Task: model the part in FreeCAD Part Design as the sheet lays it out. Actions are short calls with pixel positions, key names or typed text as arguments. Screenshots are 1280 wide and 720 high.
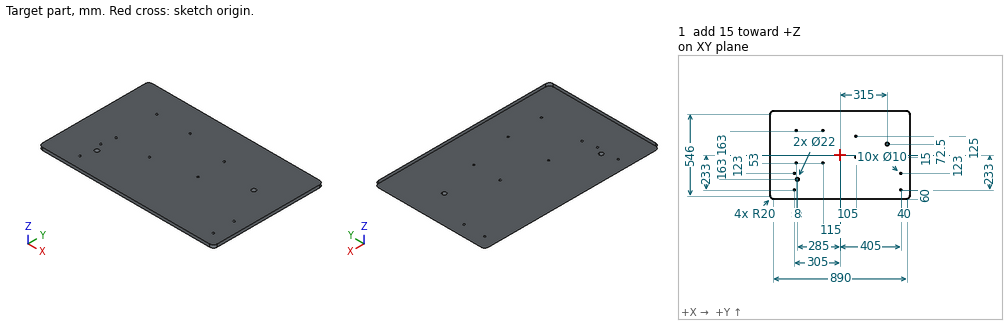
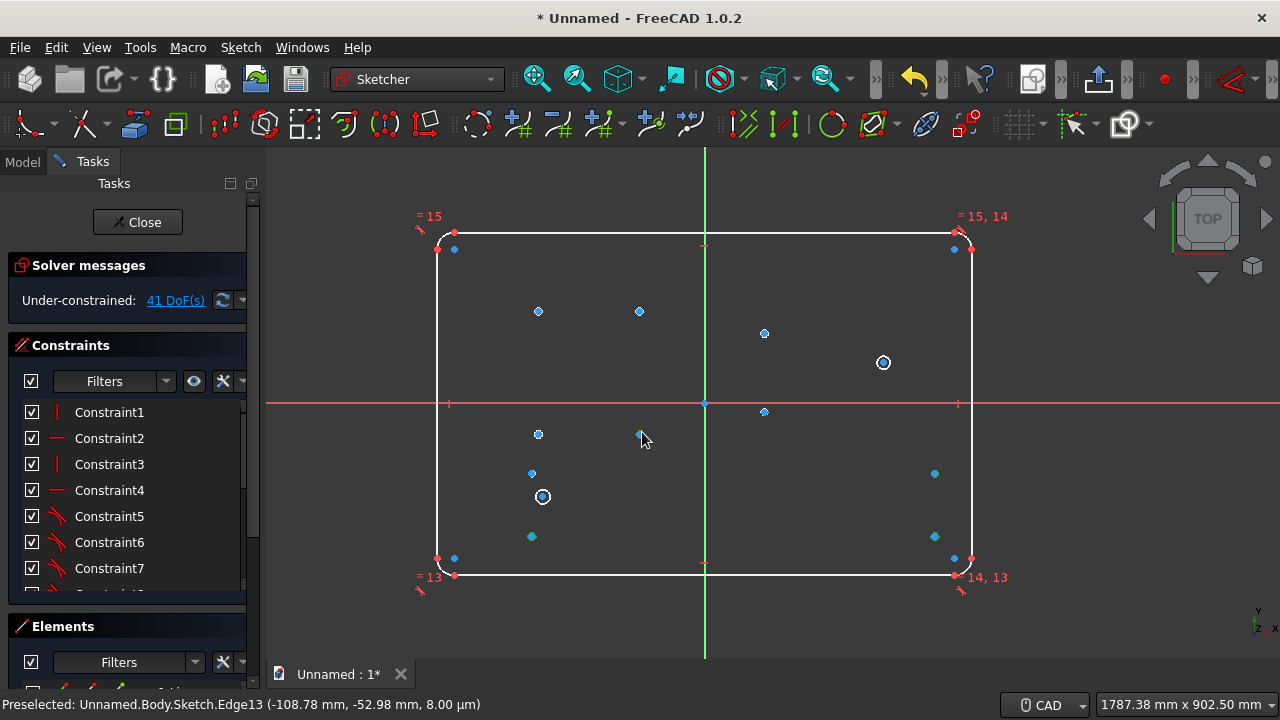
scroll(534, 471, up, 8)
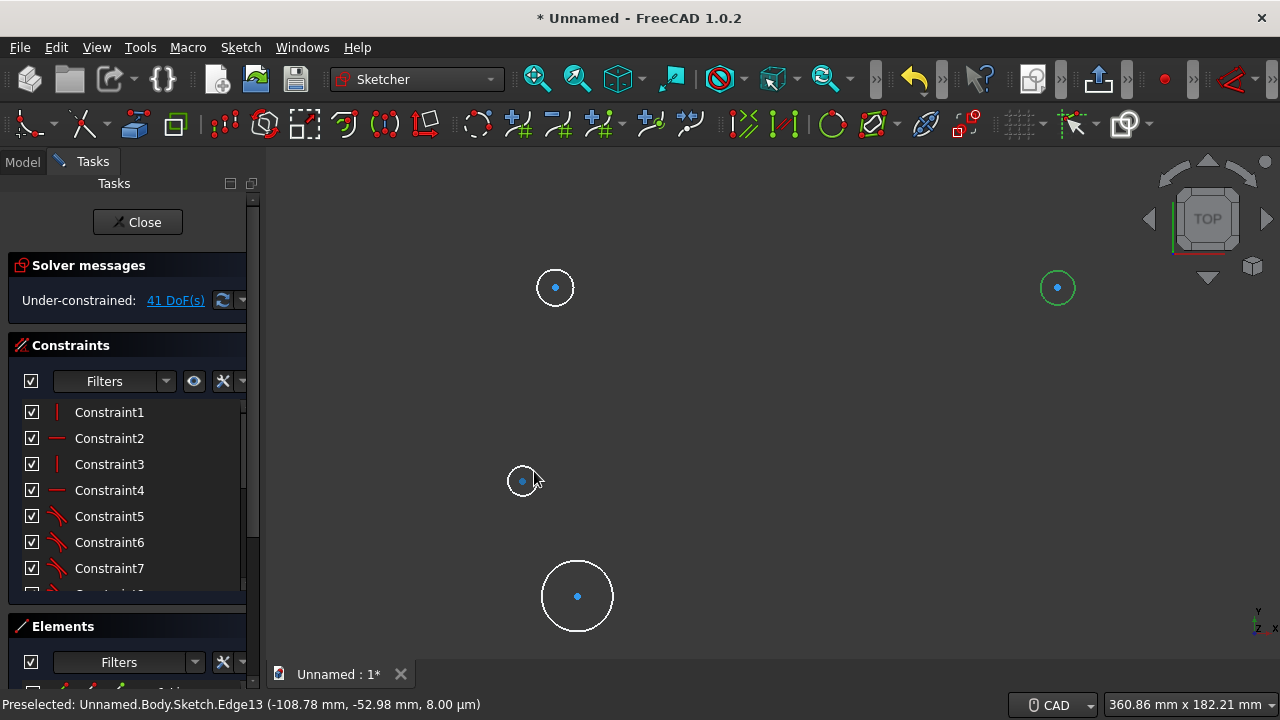
click(533, 471)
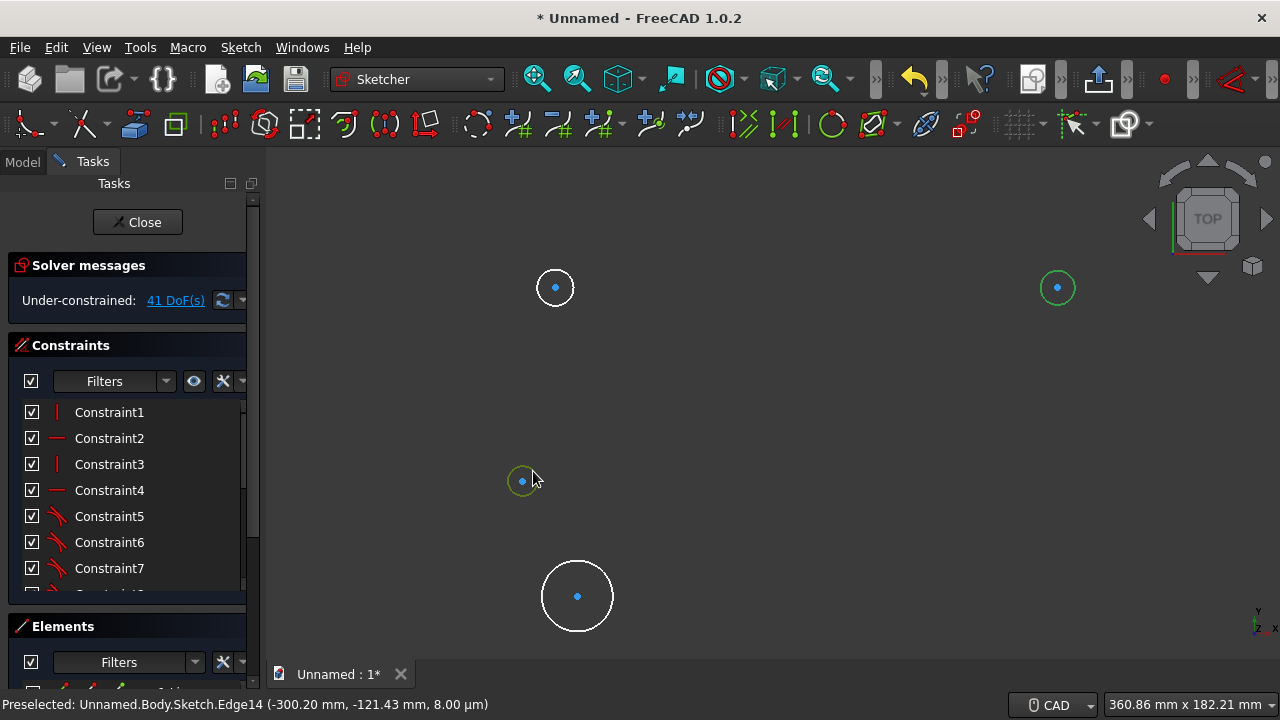
click(568, 275)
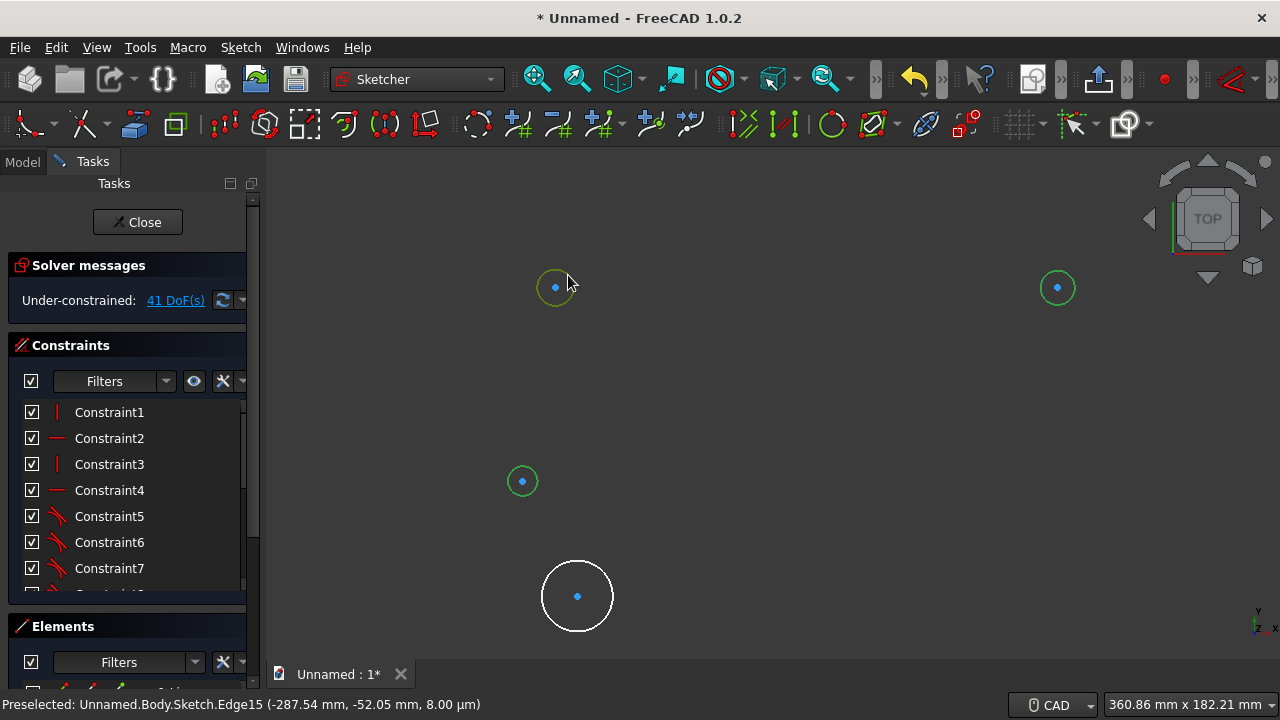
scroll(534, 471, down, 8)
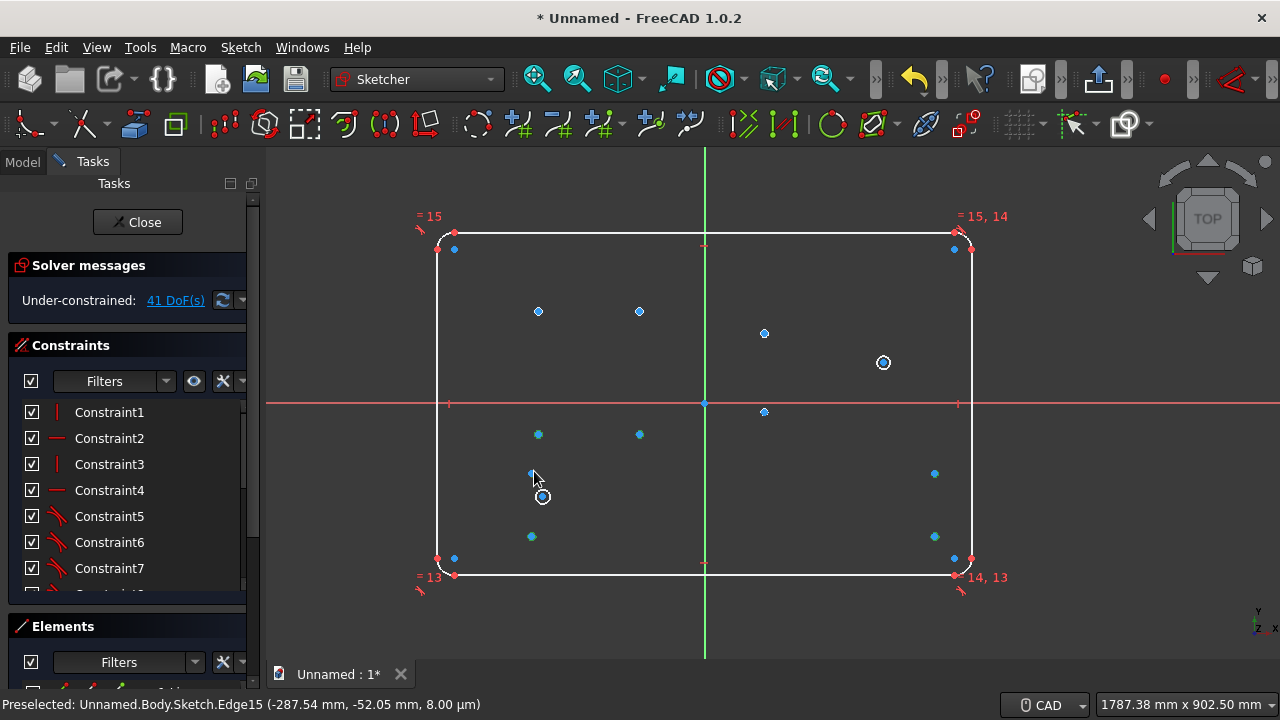
scroll(767, 410, up, 8)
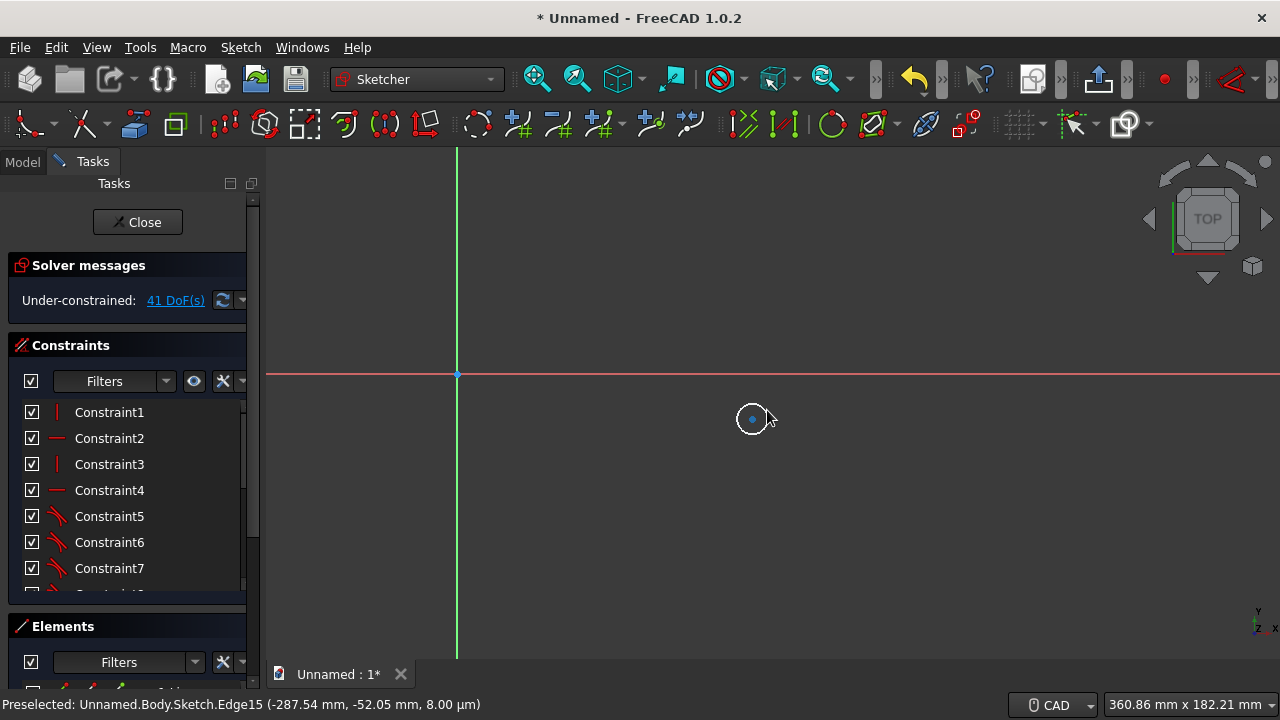
click(763, 408)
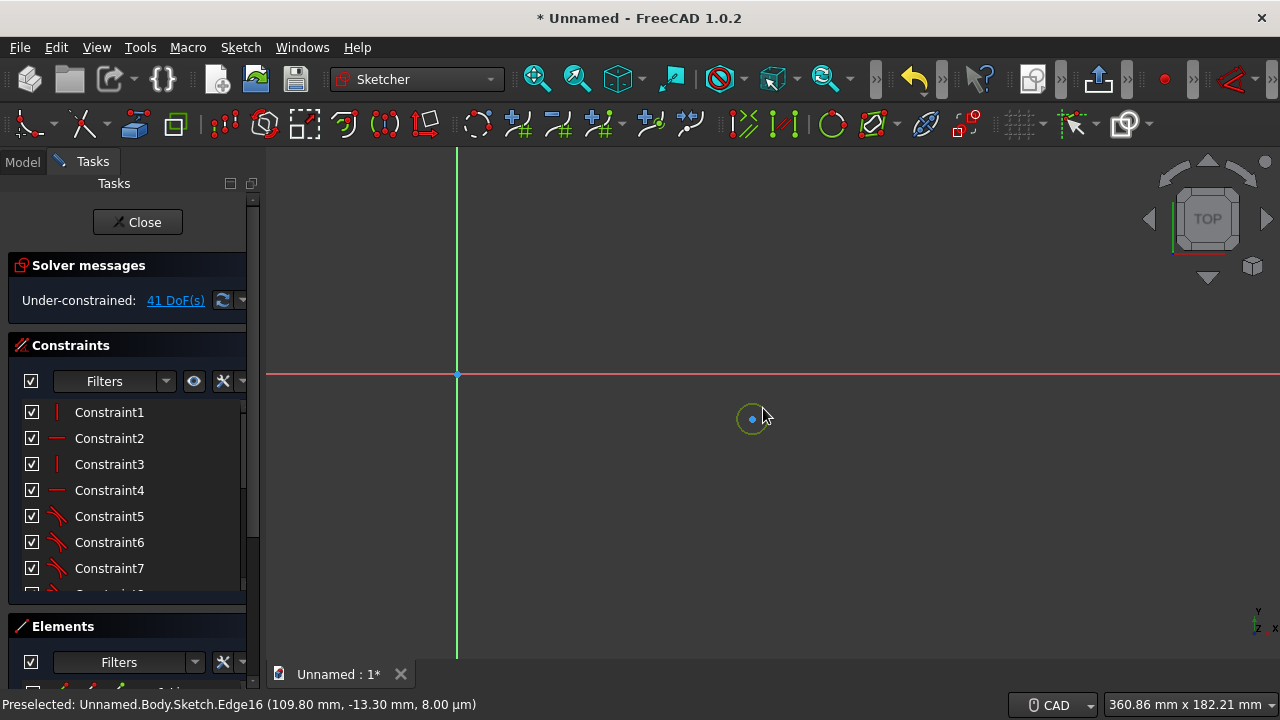
scroll(767, 410, down, 8)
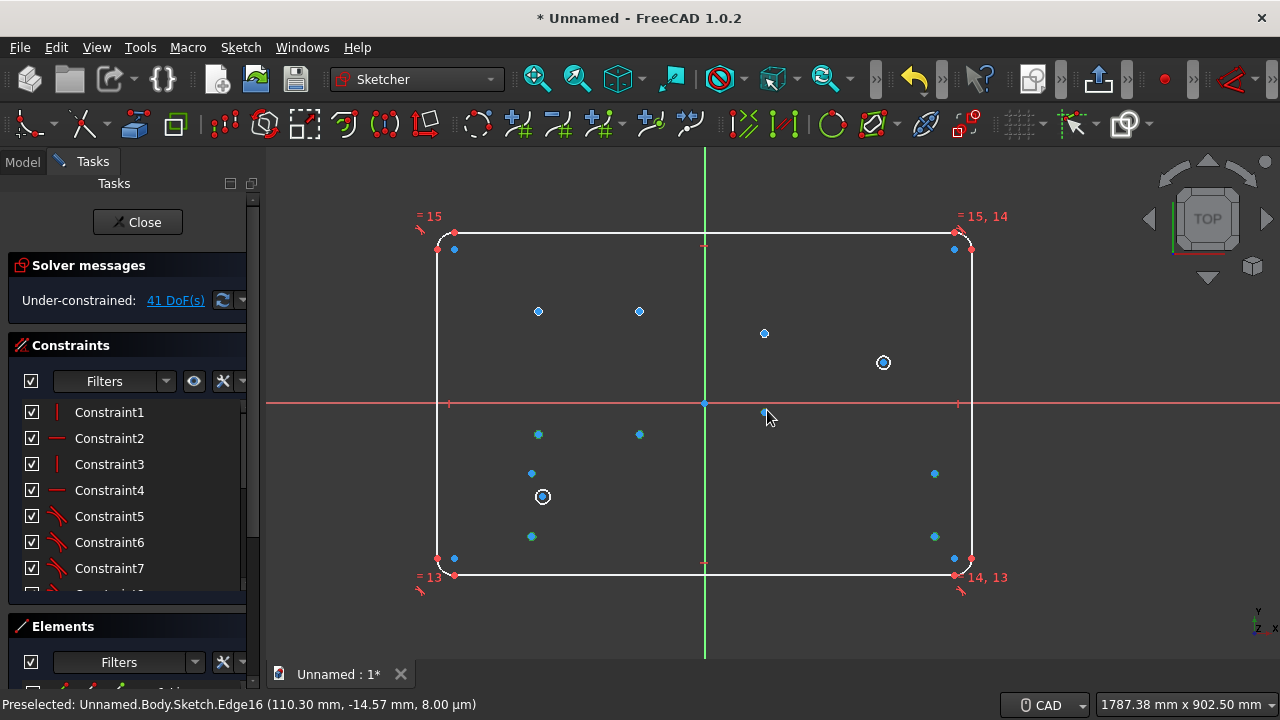
scroll(767, 331, up, 7)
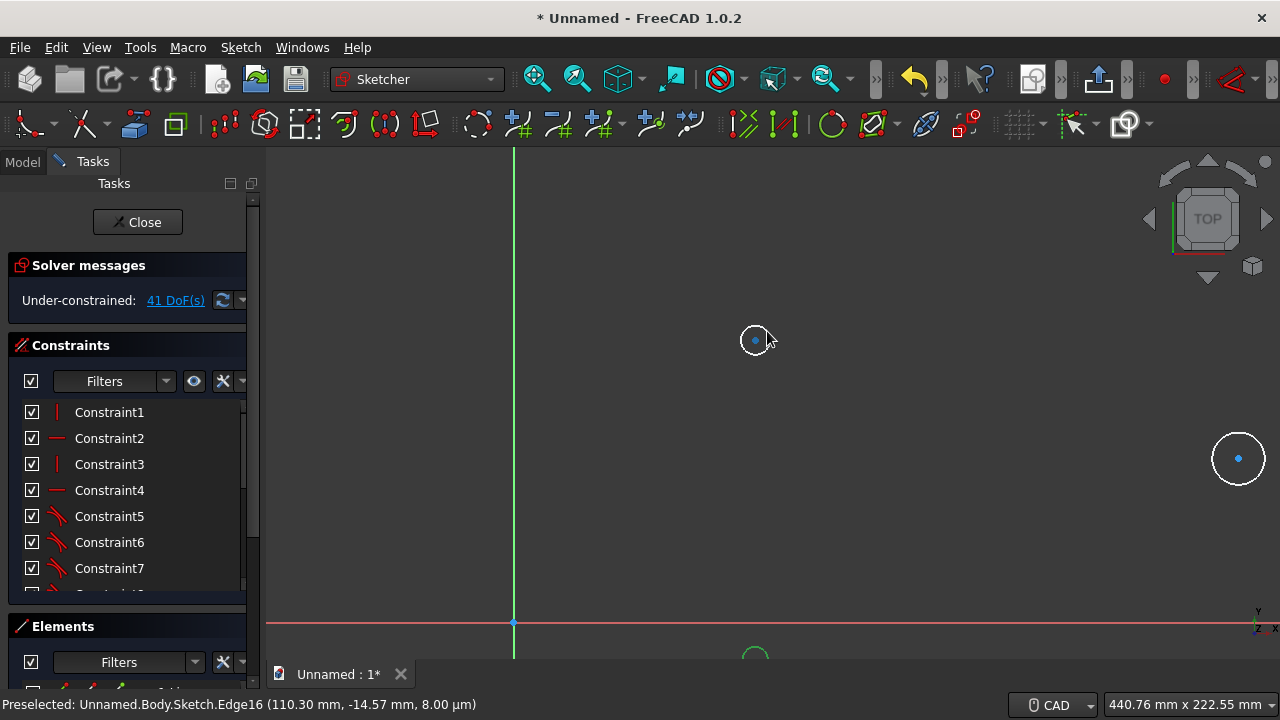
click(766, 330)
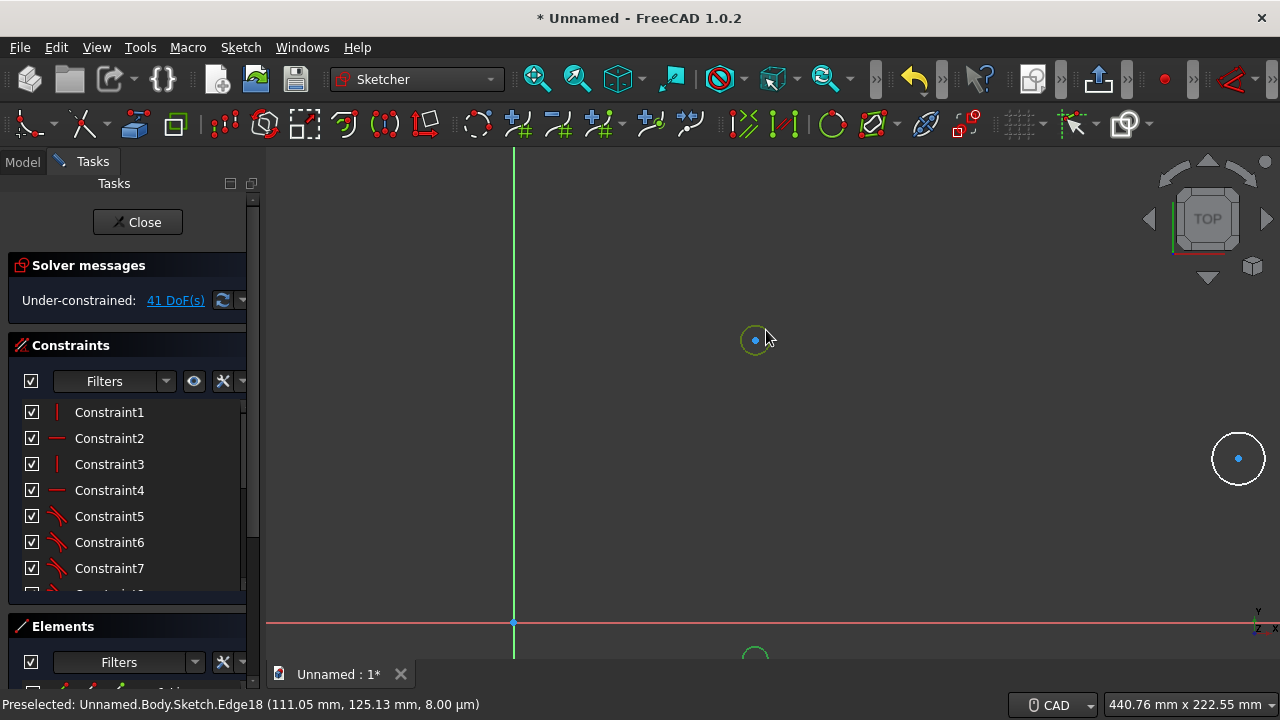
scroll(767, 331, down, 7)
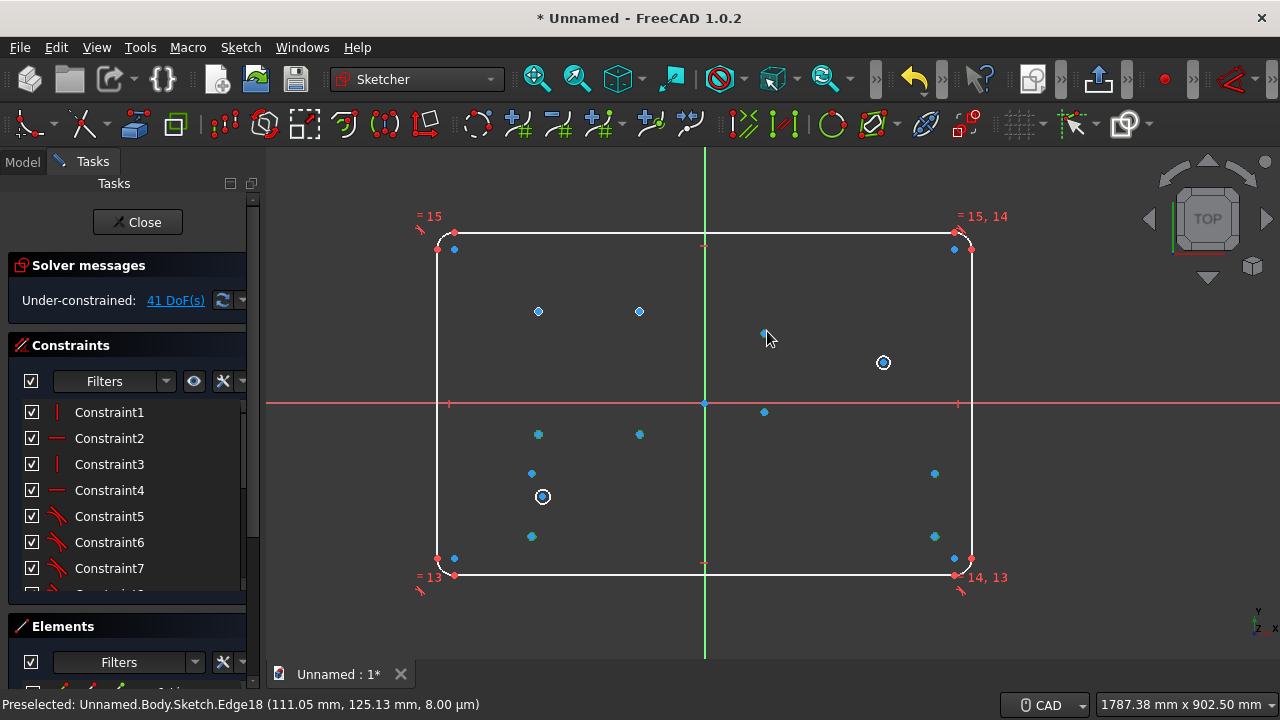
scroll(642, 309, up, 7)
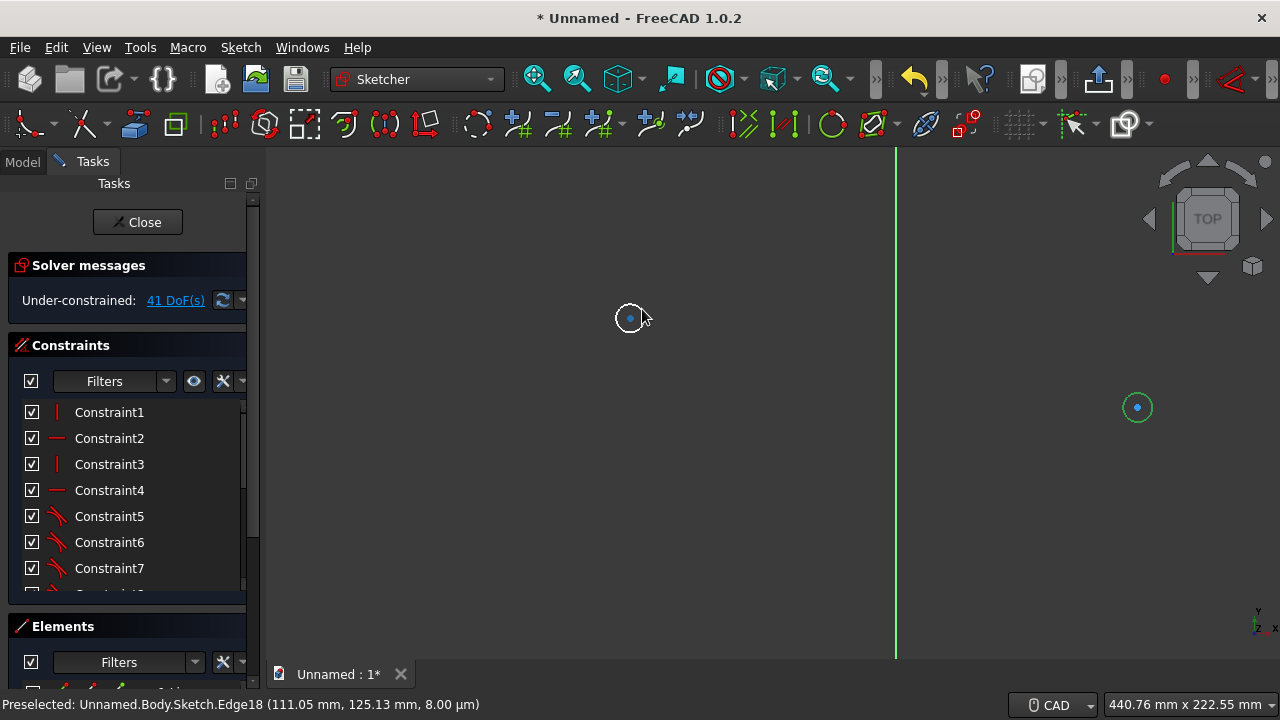
click(640, 308)